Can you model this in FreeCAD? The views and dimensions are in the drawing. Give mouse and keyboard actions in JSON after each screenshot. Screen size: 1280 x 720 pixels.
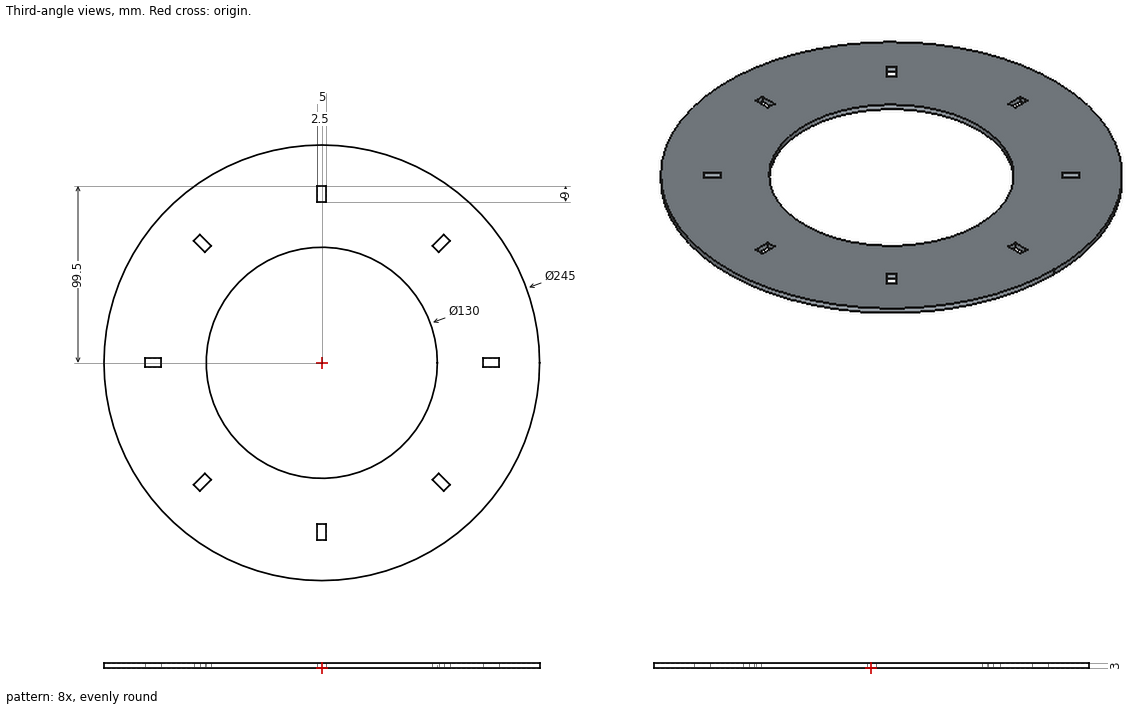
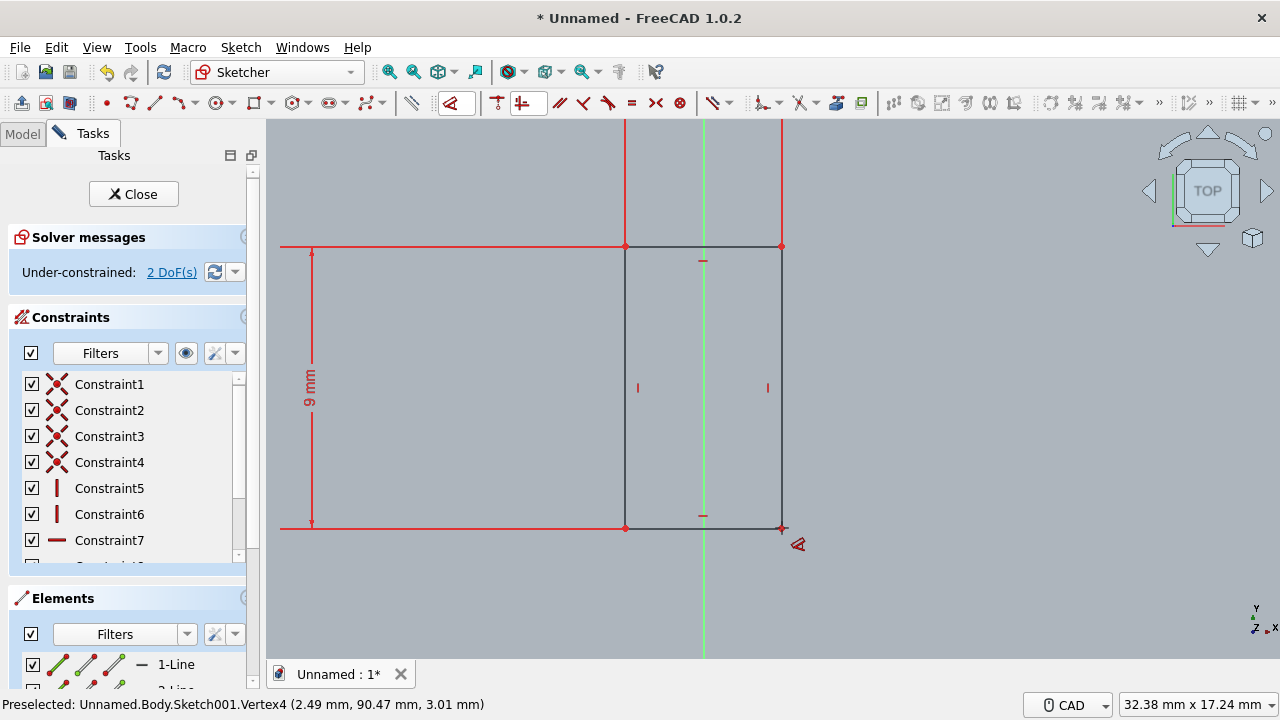
{"action": "left_click", "coordinate": [625, 247]}
{"action": "left_click", "coordinate": [664, 213]}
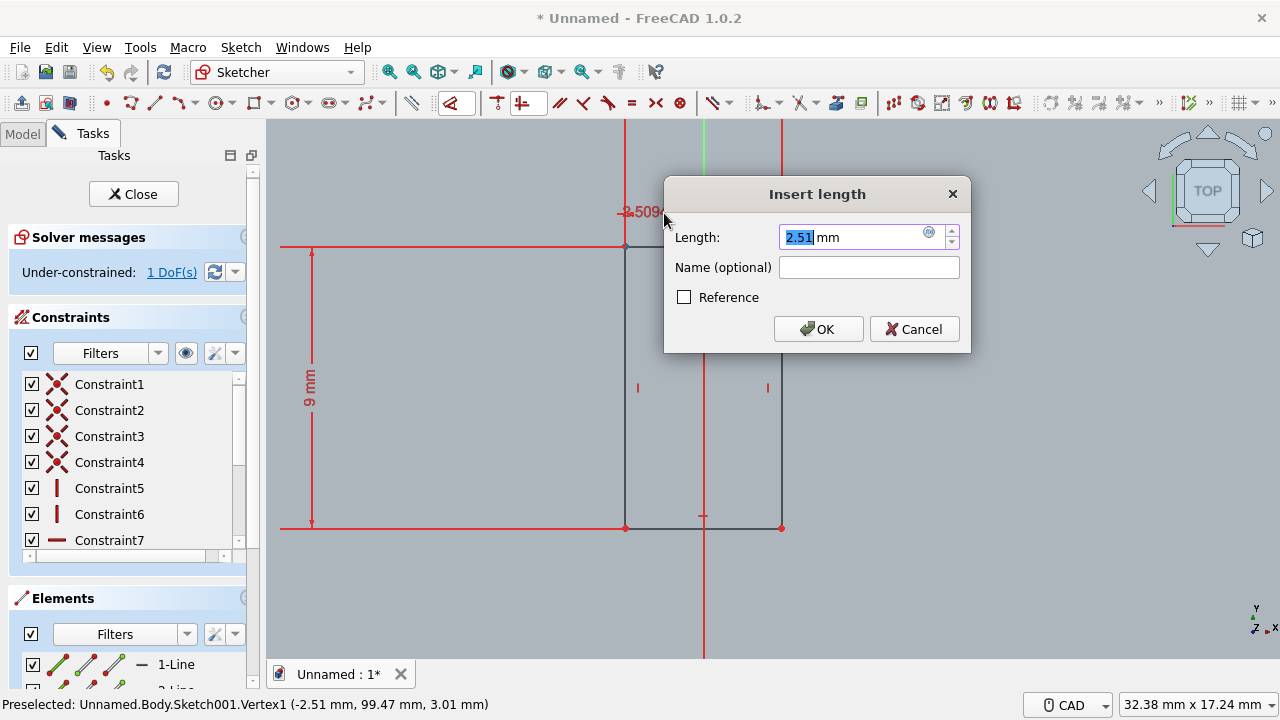
{"action": "type", "text": "2.5"}
{"action": "key", "text": "Return"}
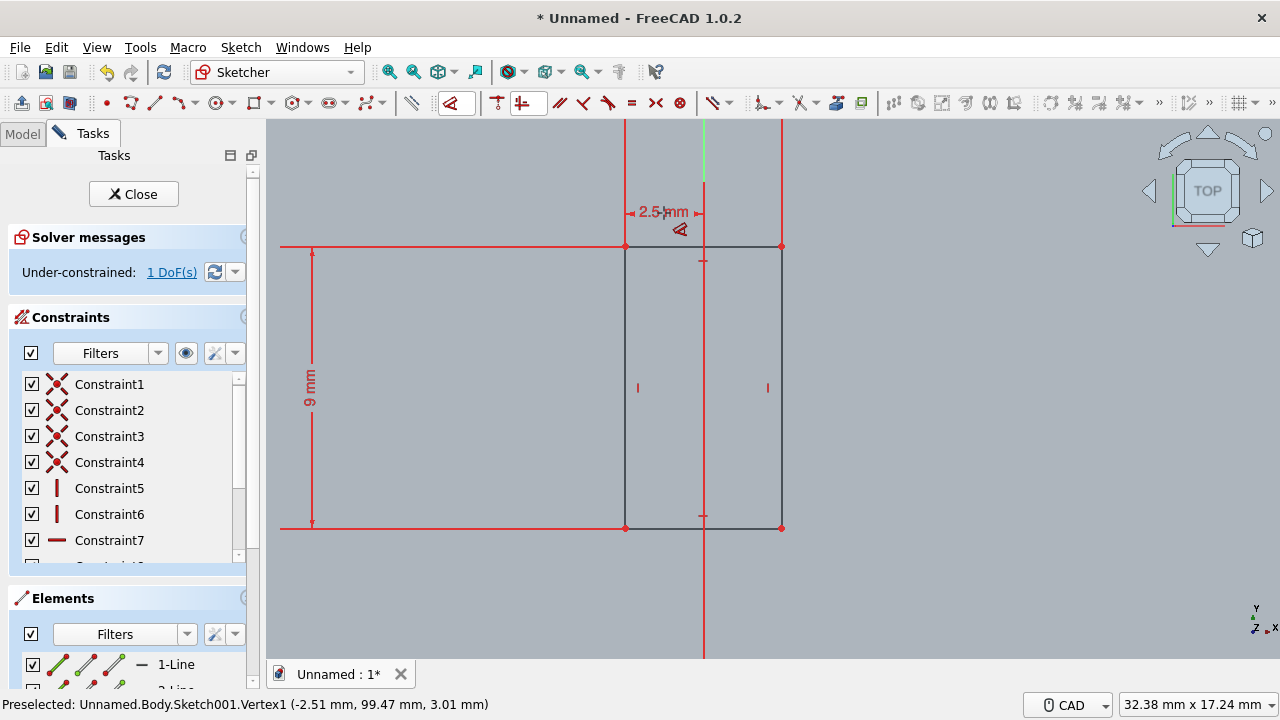
{"action": "left_click", "coordinate": [625, 247]}
{"action": "left_click", "coordinate": [591, 439]}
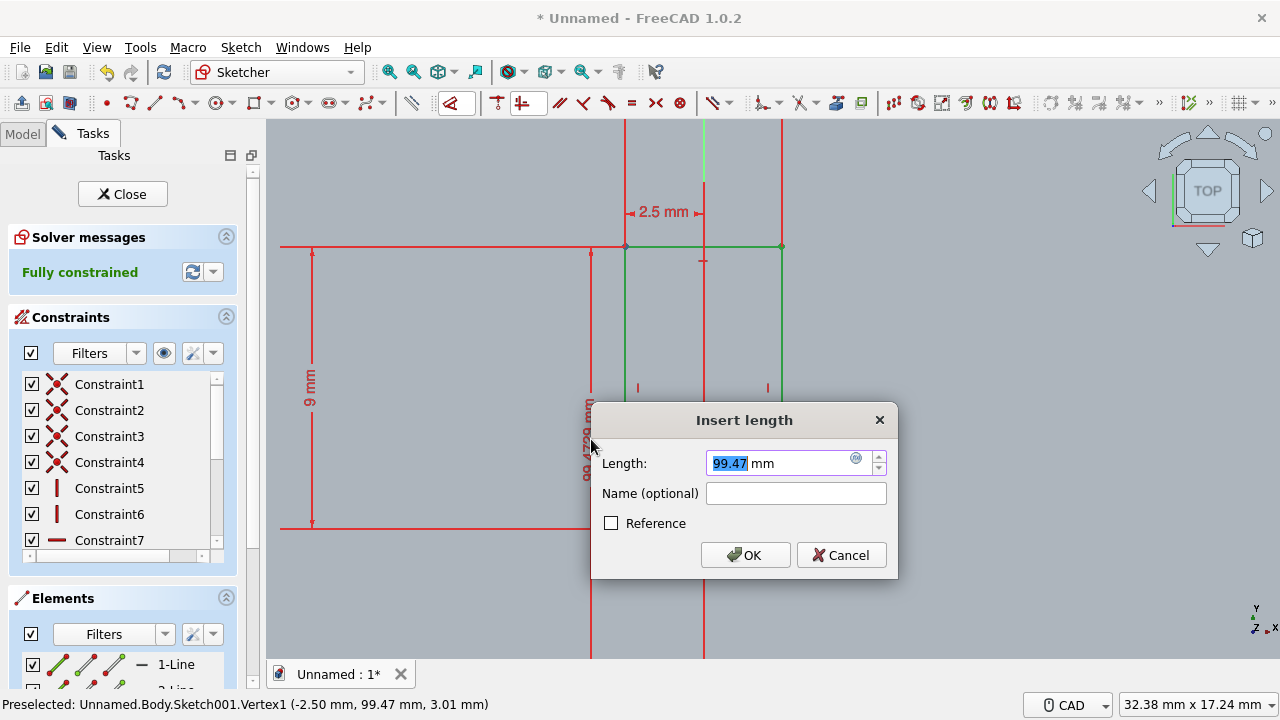
{"action": "type", "text": "99.5"}
{"action": "key", "text": "Return"}
{"action": "key", "text": "Escape"}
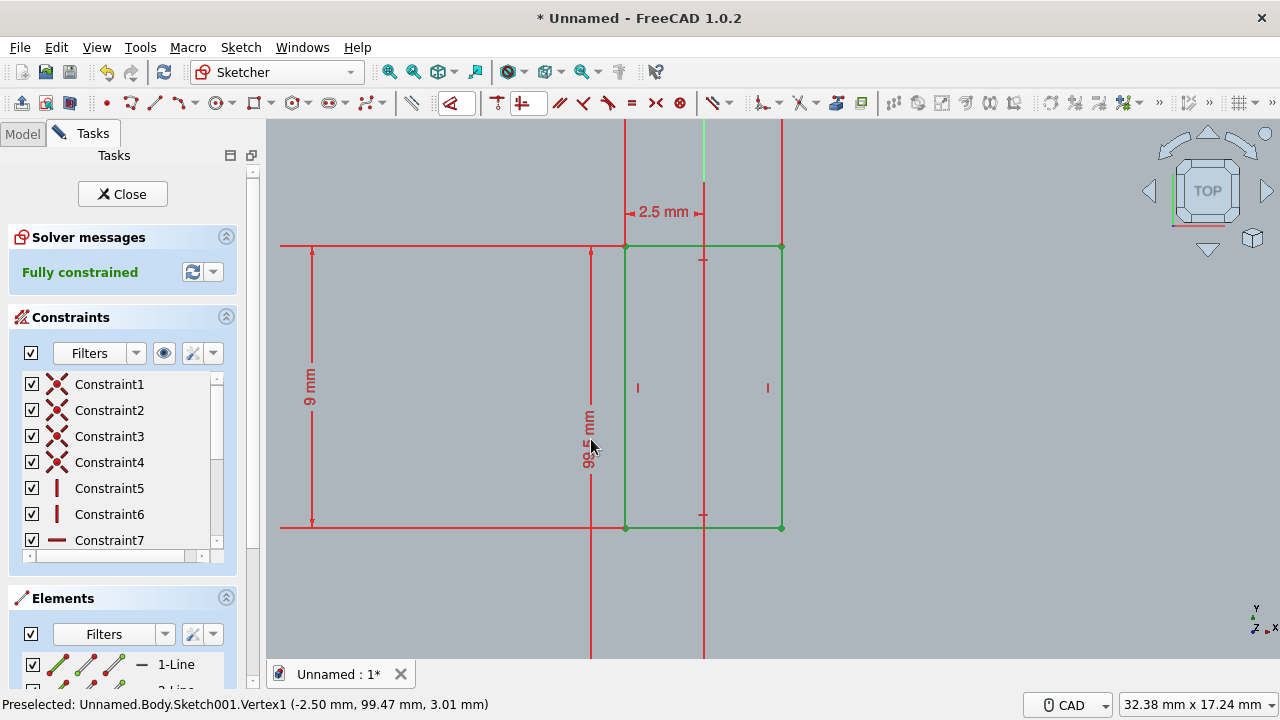
{"action": "left_click", "coordinate": [123, 194]}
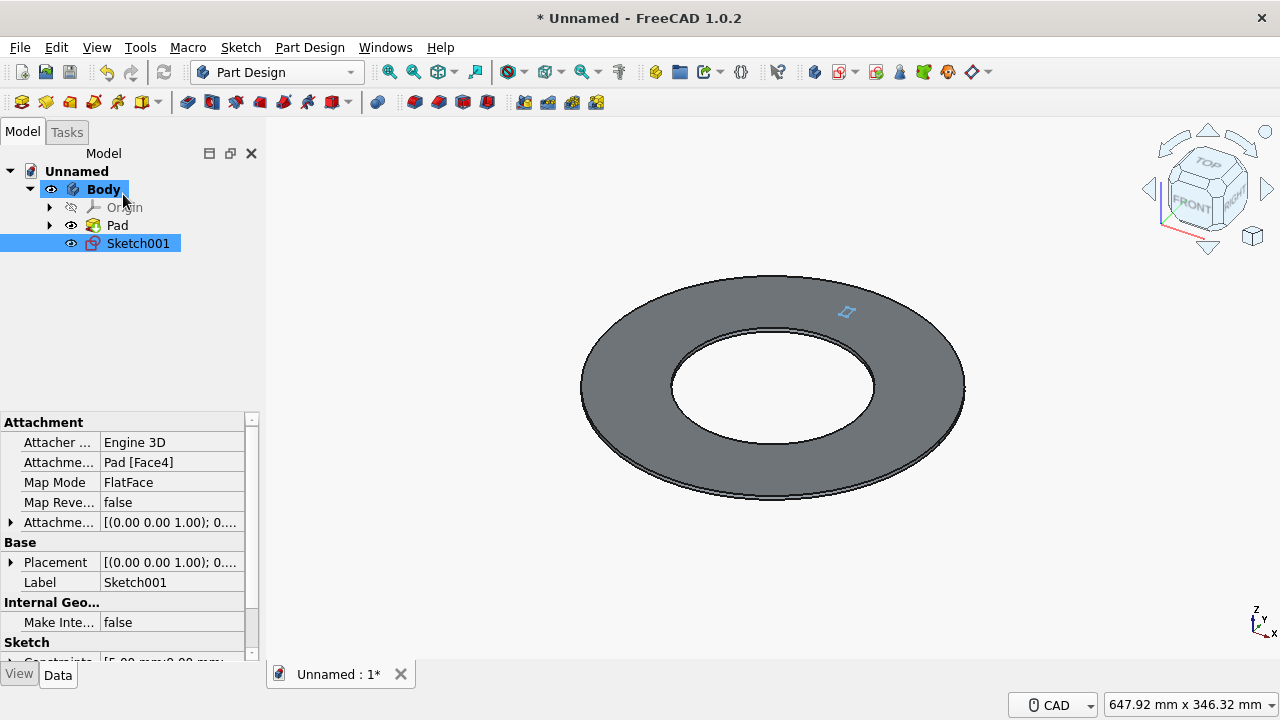
{"action": "left_click", "coordinate": [188, 102]}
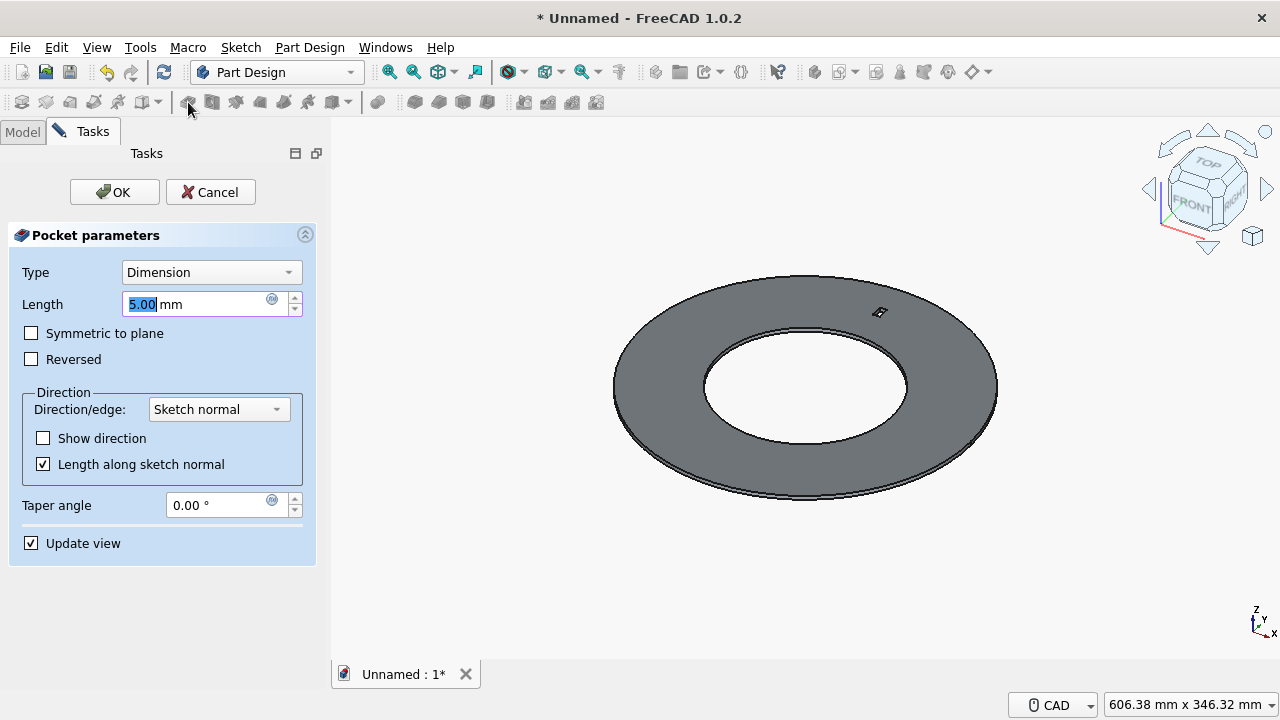
{"action": "type", "text": "5"}
{"action": "key", "text": "Tab"}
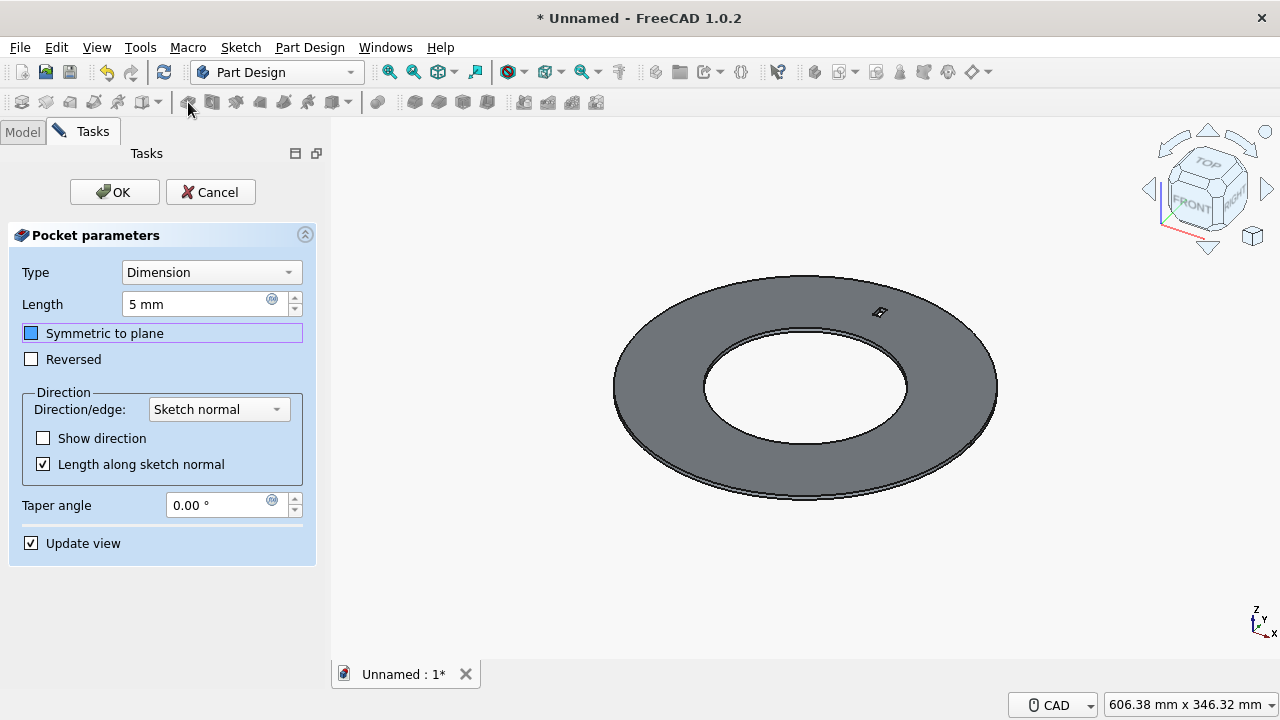
{"action": "left_click", "coordinate": [115, 192]}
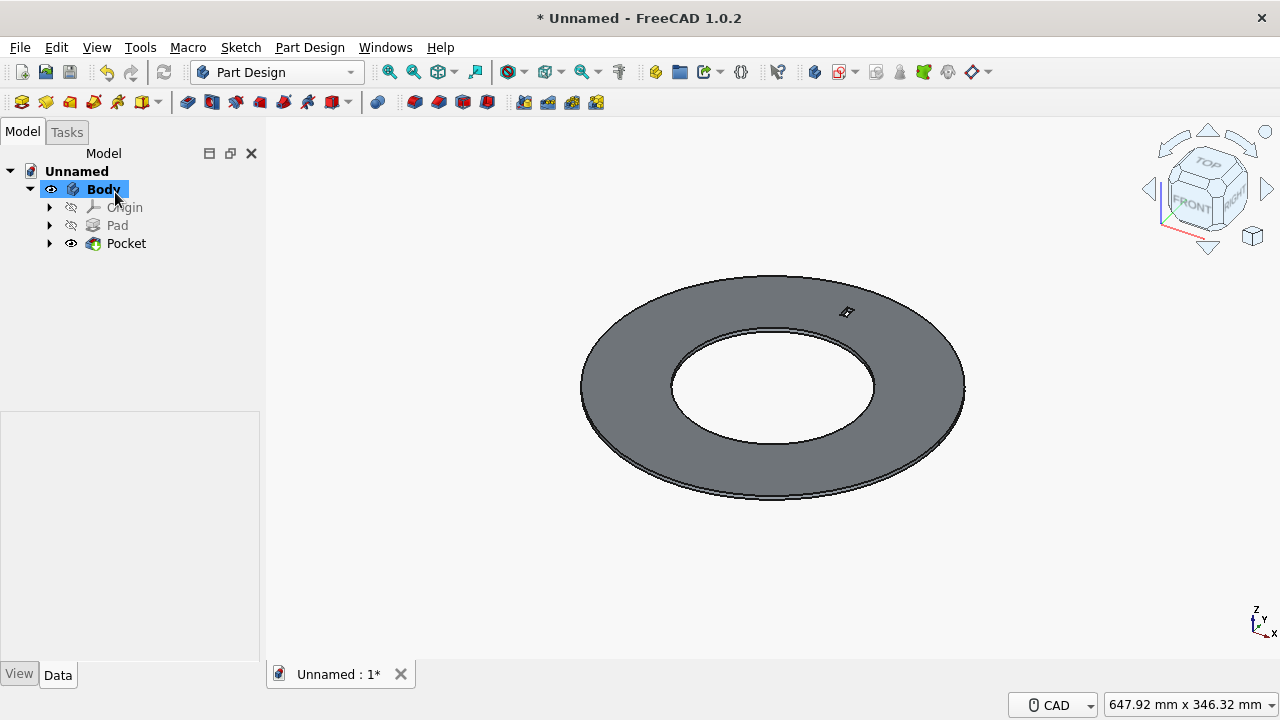
{"action": "left_click", "coordinate": [116, 243]}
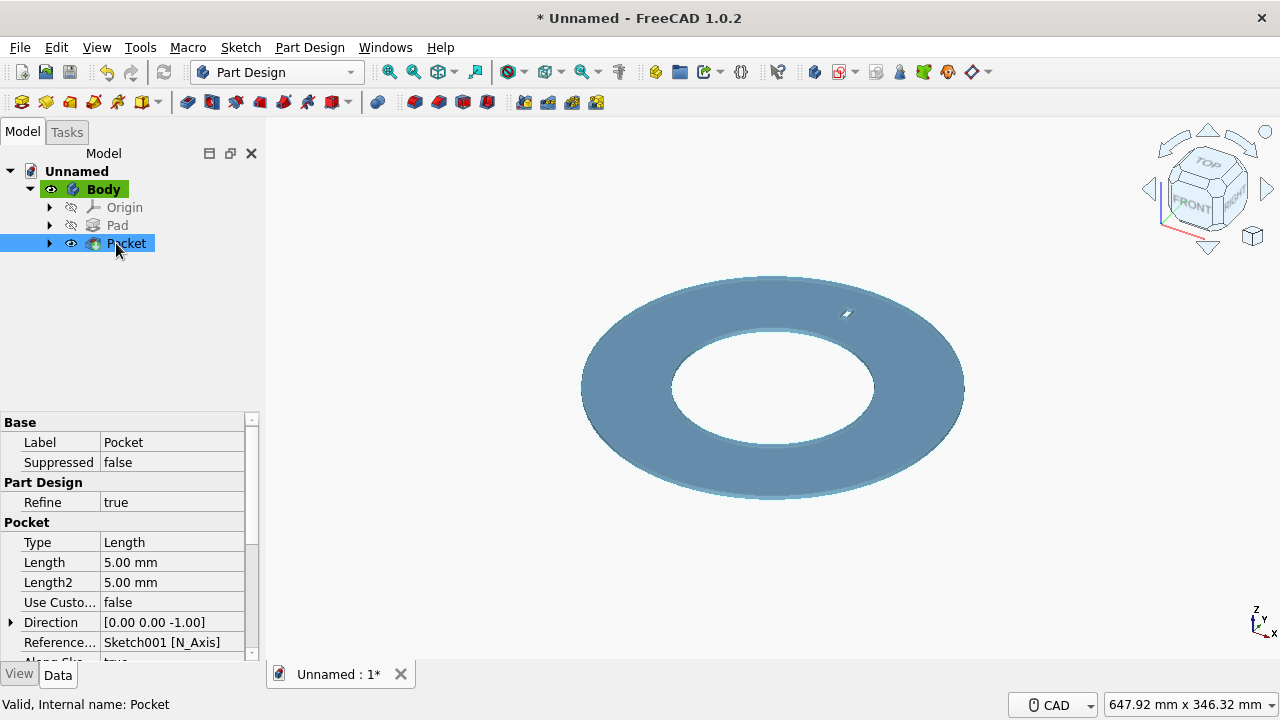
{"action": "left_click", "coordinate": [572, 102]}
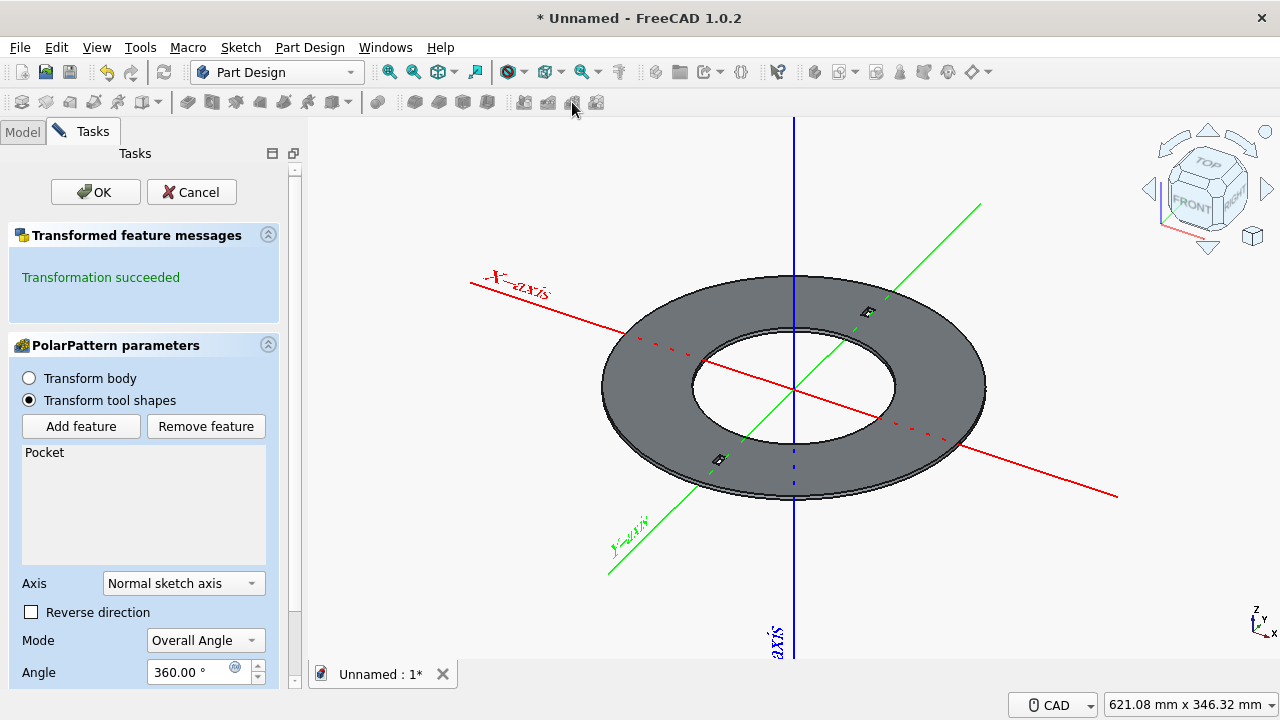
{"action": "left_click", "coordinate": [184, 584]}